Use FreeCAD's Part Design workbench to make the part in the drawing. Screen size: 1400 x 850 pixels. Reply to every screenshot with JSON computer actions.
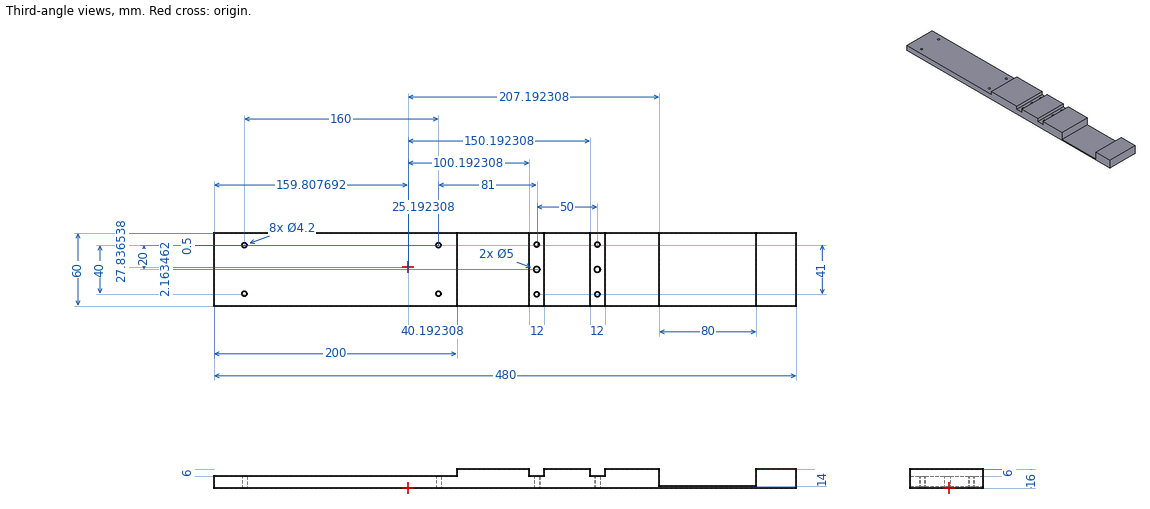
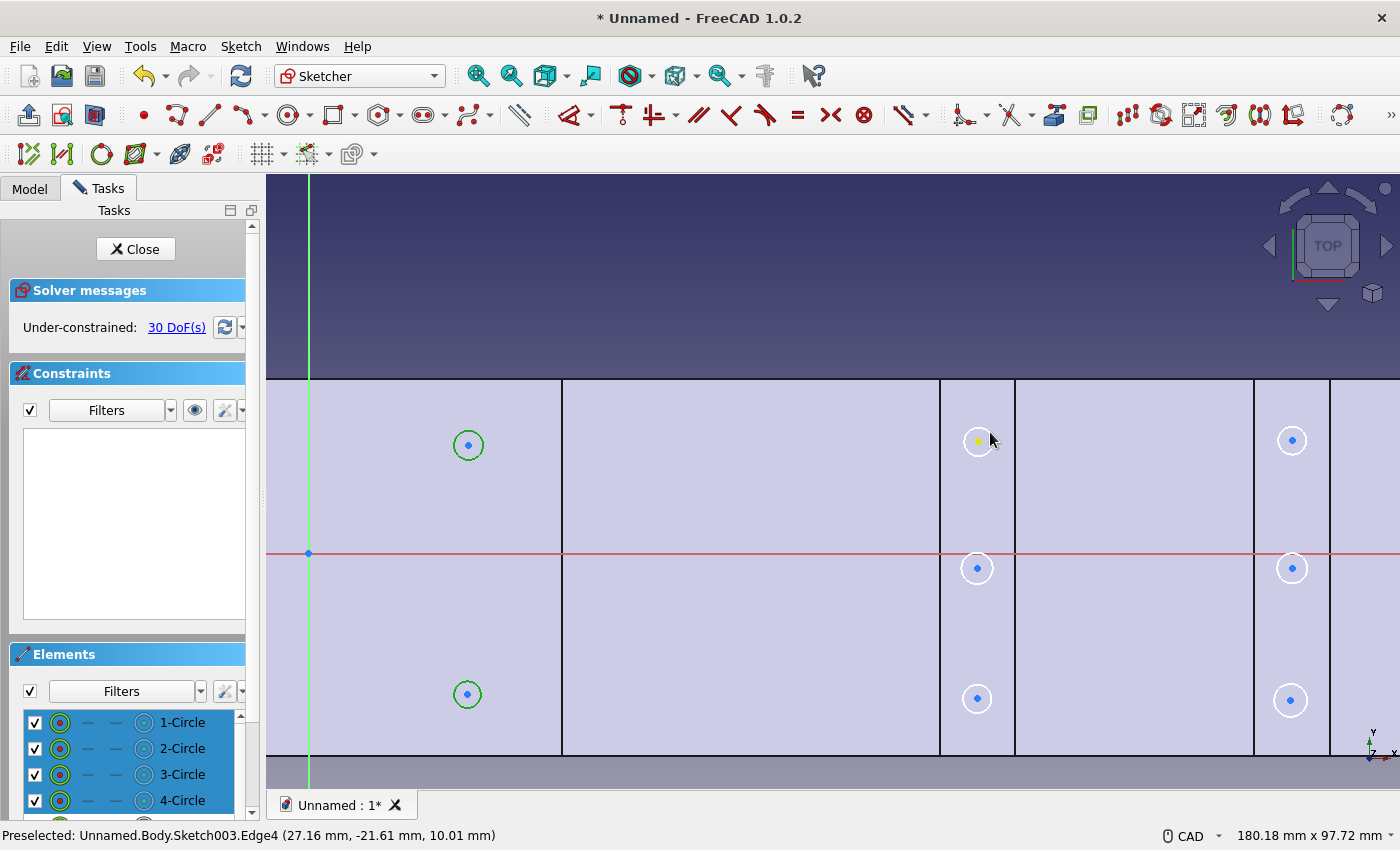
{"action": "left_click", "coordinate": [989, 432]}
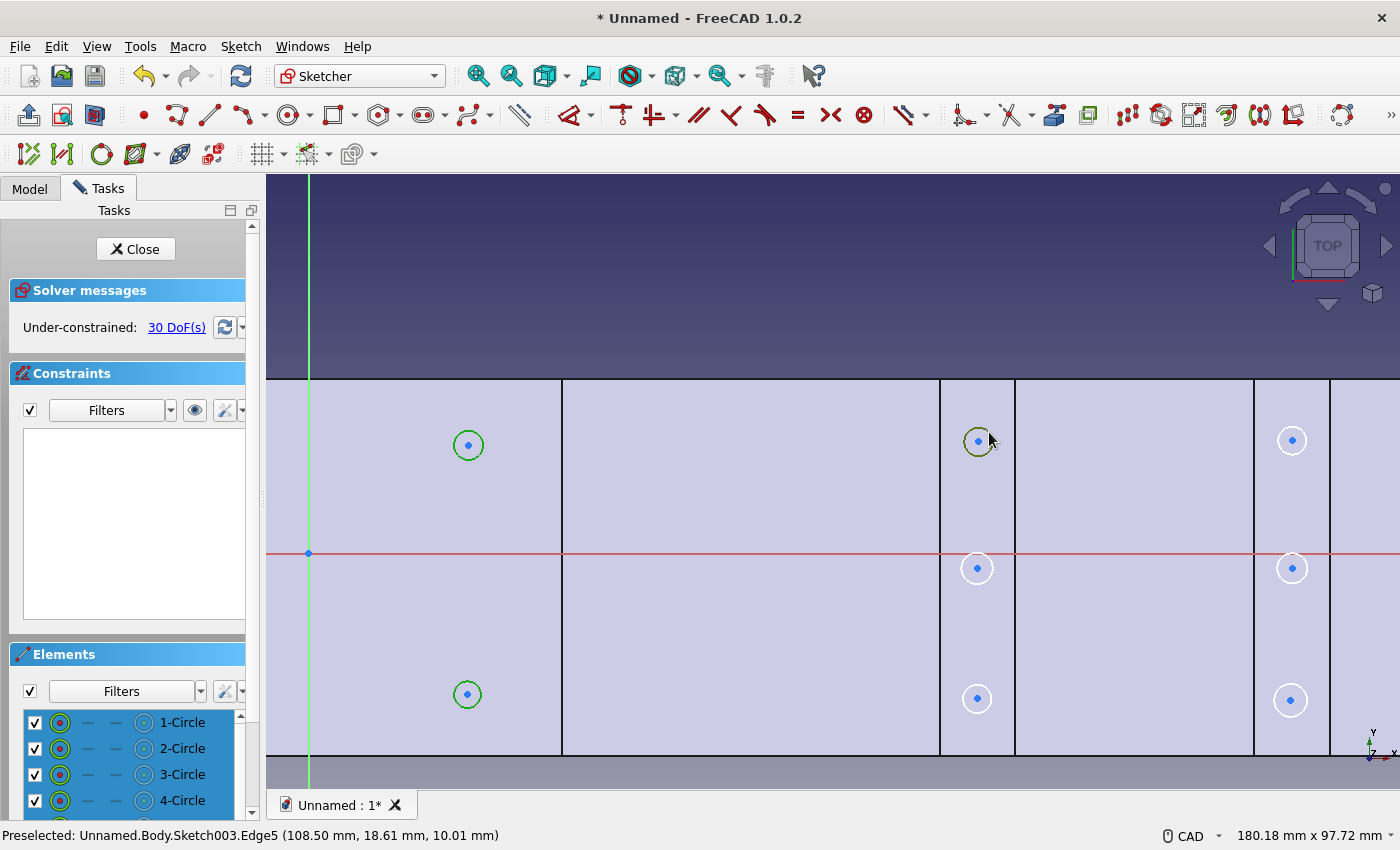
{"action": "left_click", "coordinate": [987, 689]}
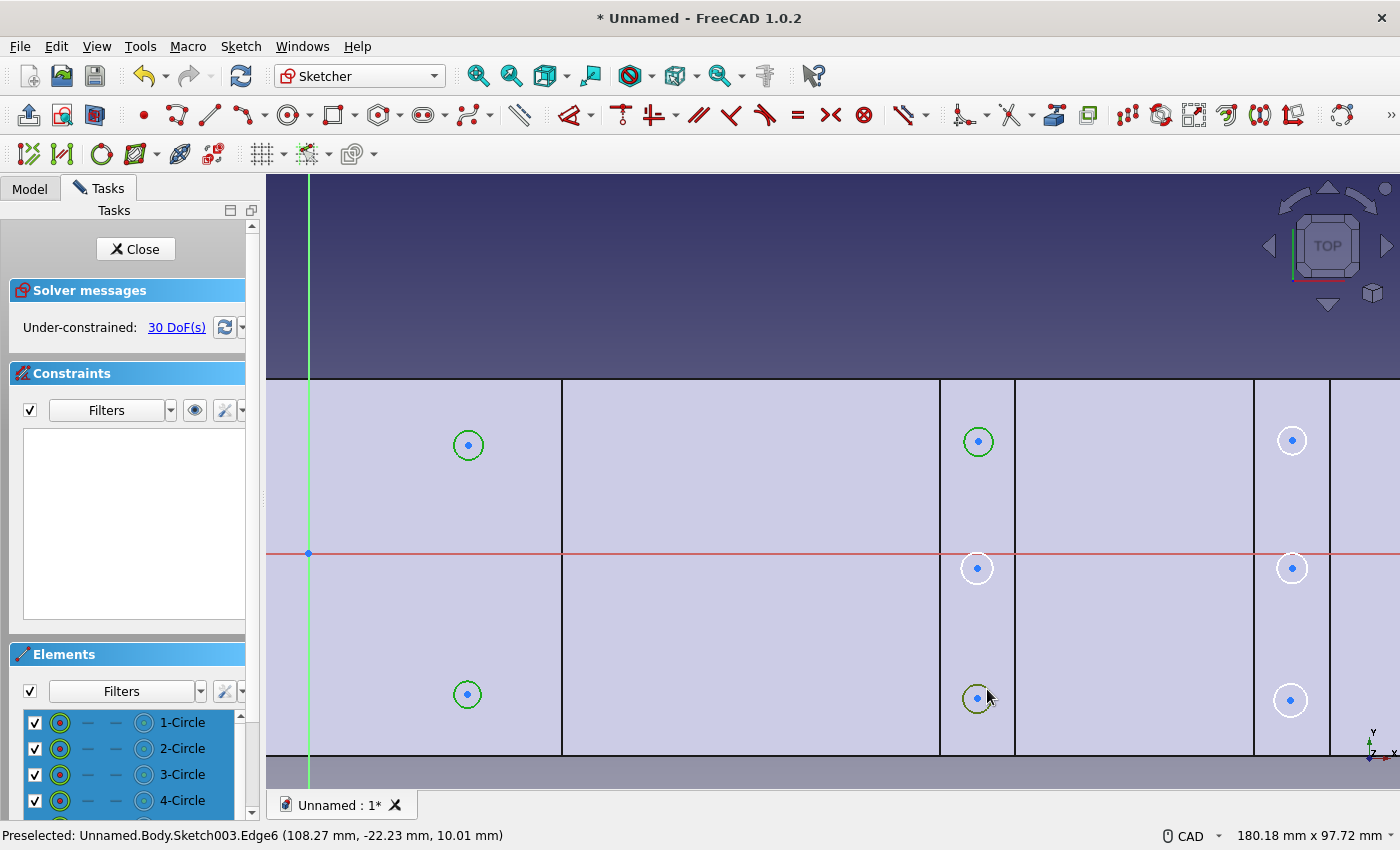
{"action": "scroll", "coordinate": [990, 432], "scroll_direction": "down", "scroll_amount": 5}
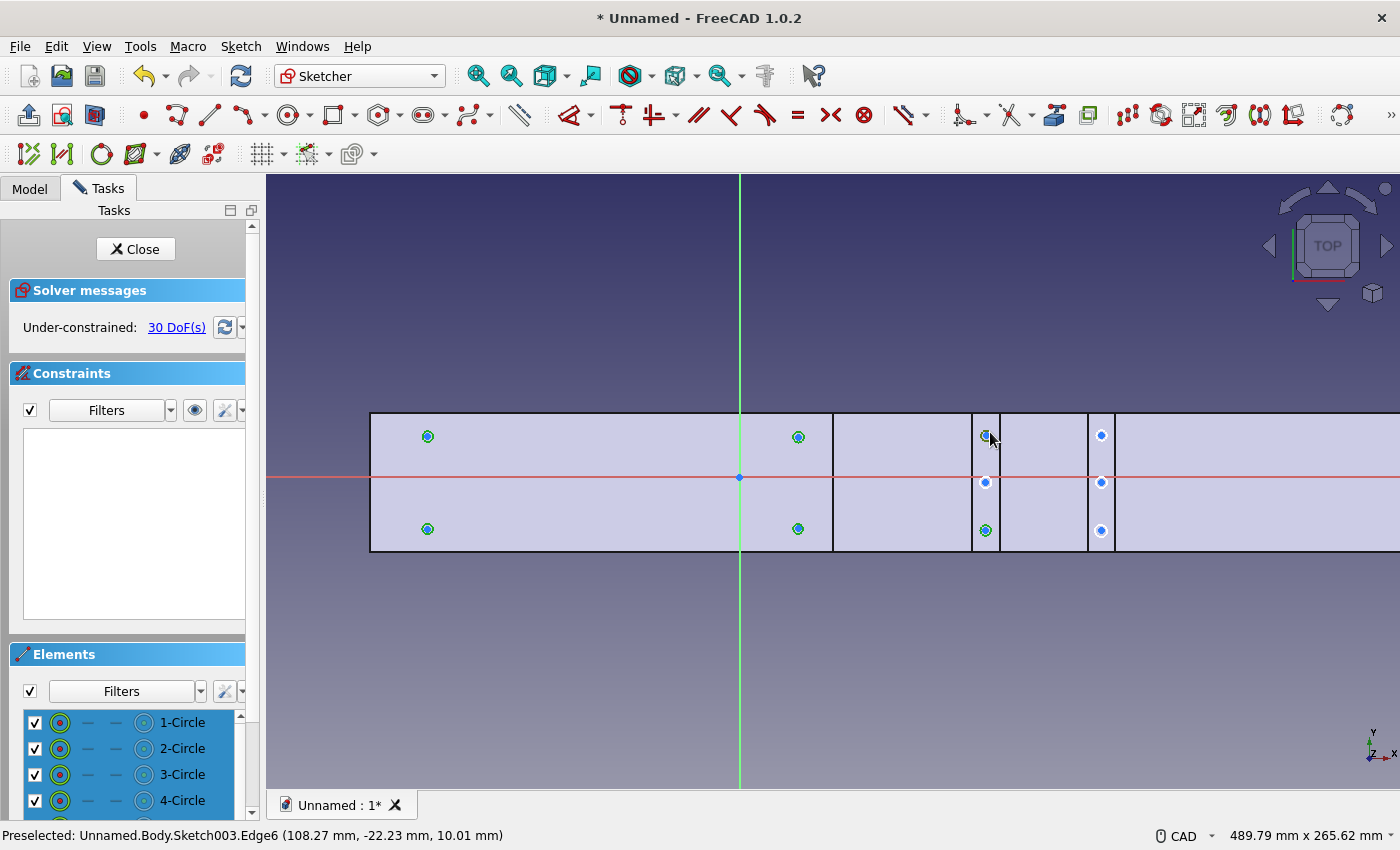
{"action": "scroll", "coordinate": [1105, 432], "scroll_direction": "up", "scroll_amount": 5}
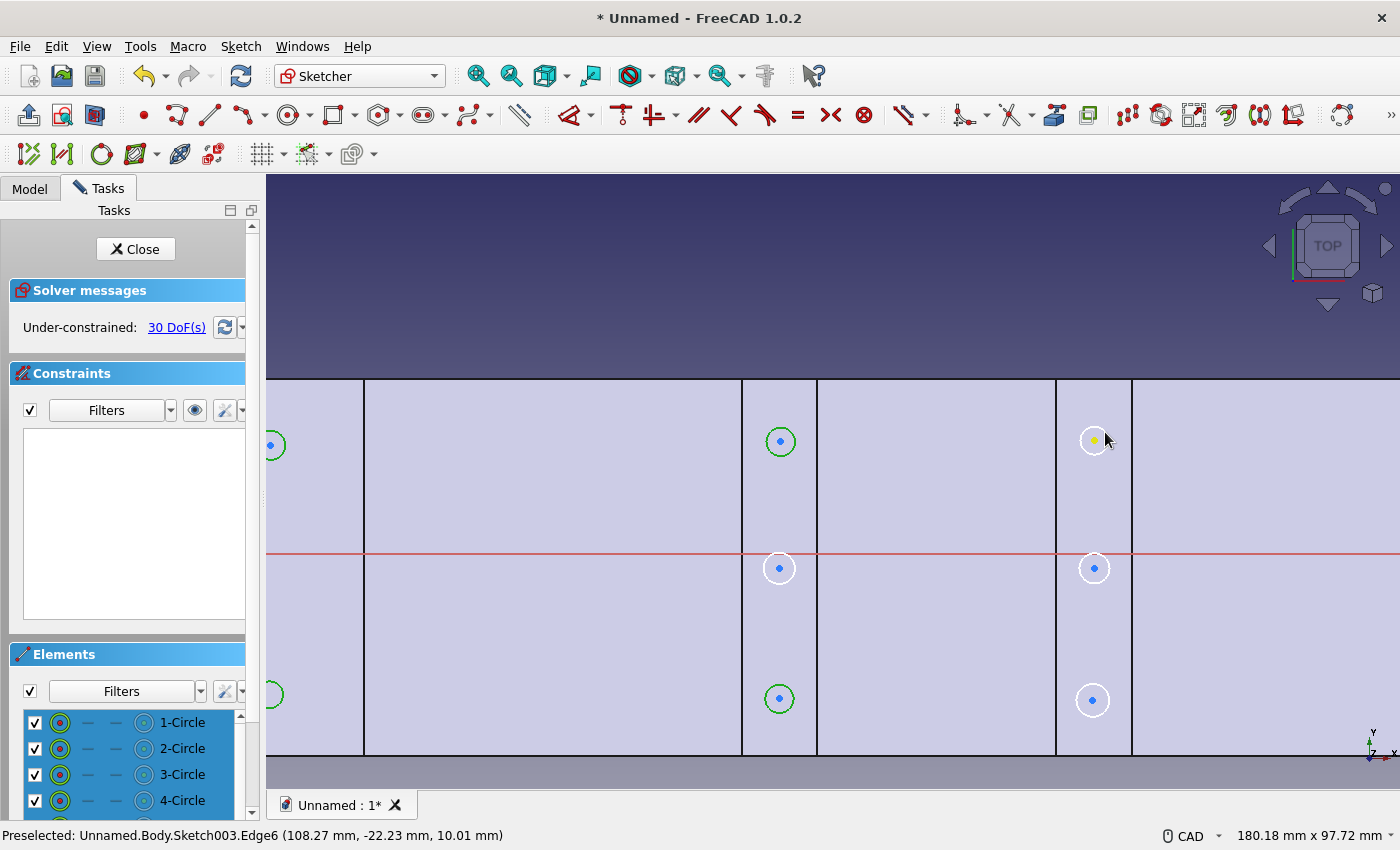
{"action": "left_click", "coordinate": [1104, 431]}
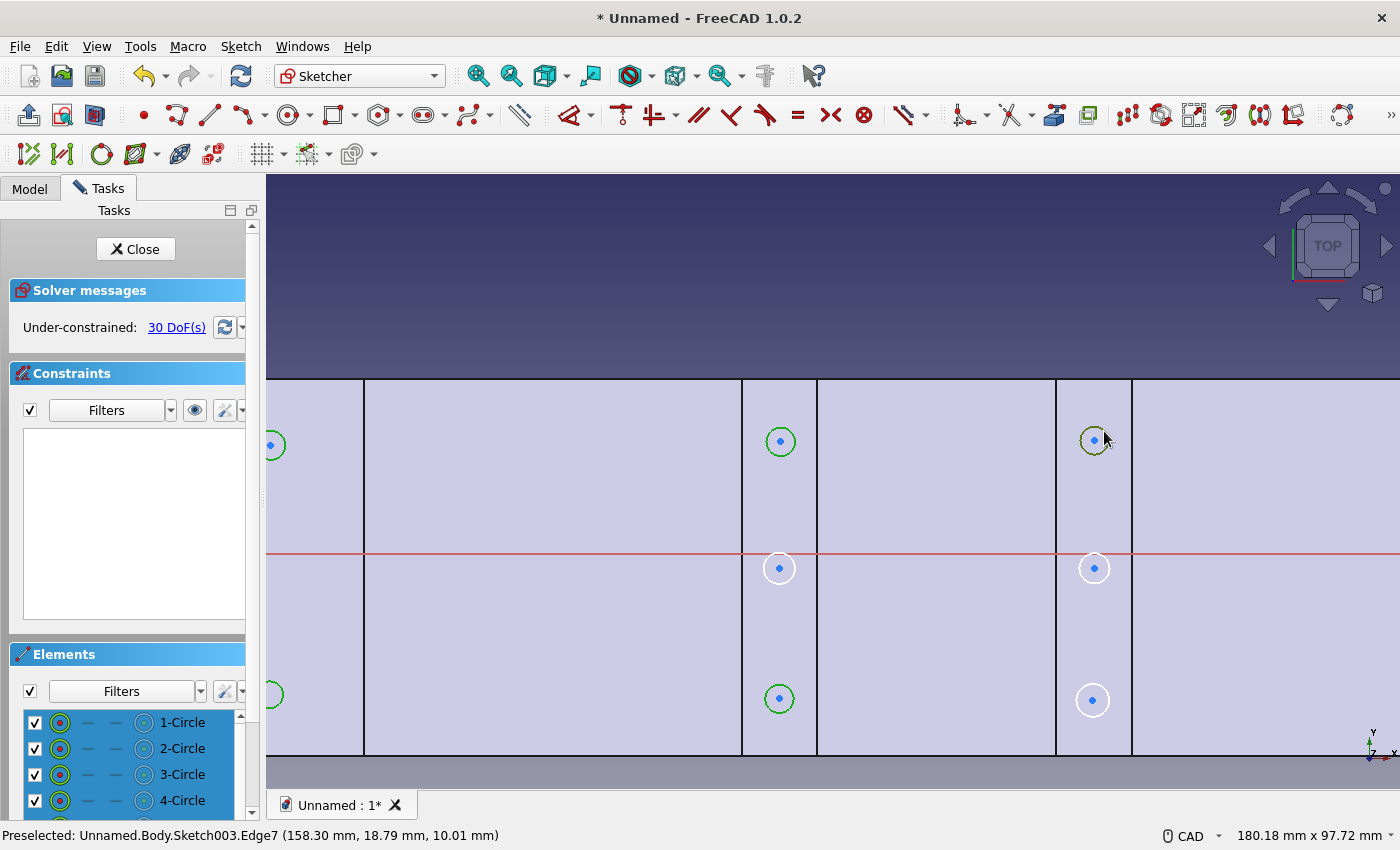
{"action": "left_click", "coordinate": [1104, 689]}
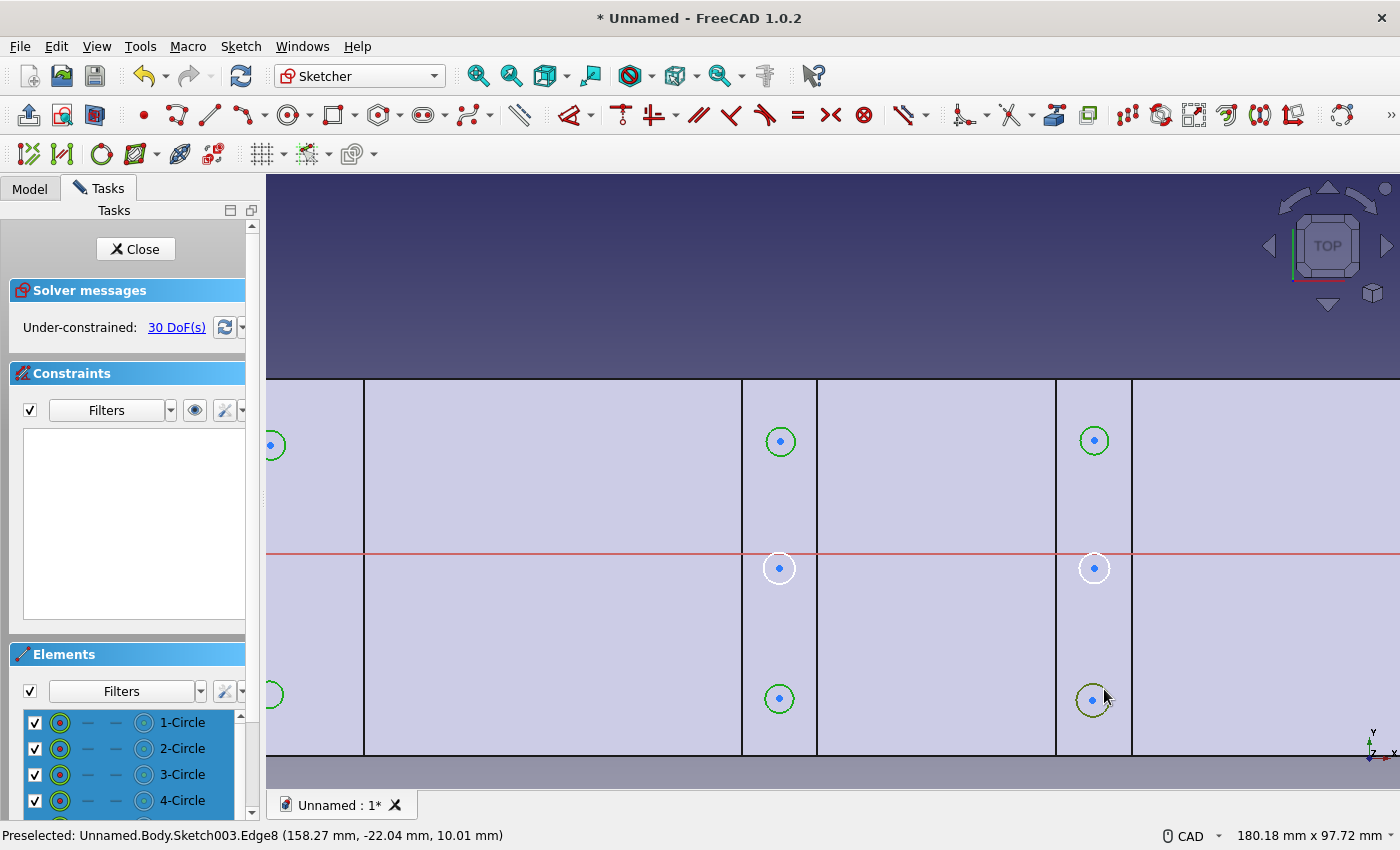
{"action": "key", "text": "e"}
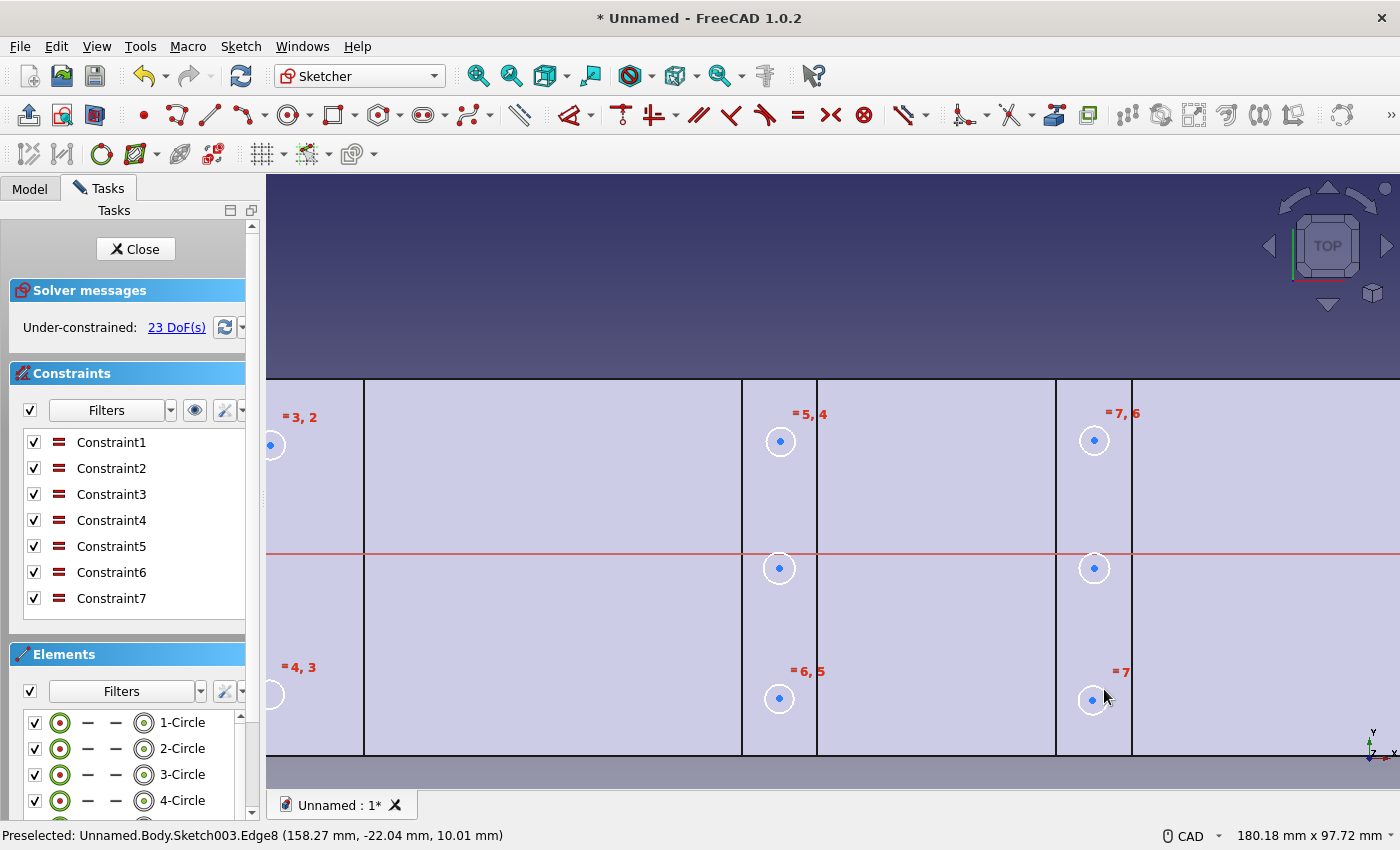
{"action": "left_click", "coordinate": [790, 557]}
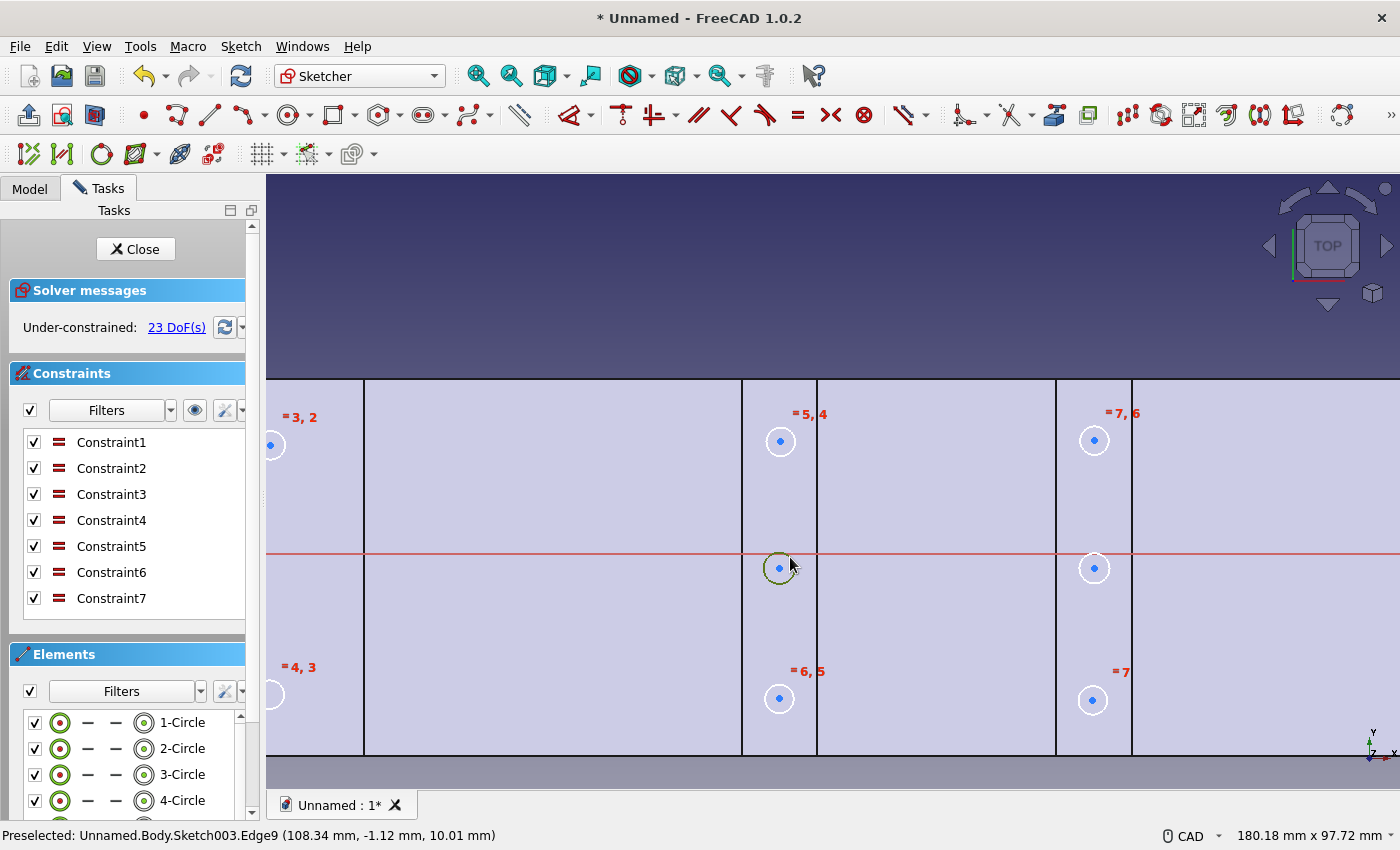
{"action": "left_click", "coordinate": [1105, 558]}